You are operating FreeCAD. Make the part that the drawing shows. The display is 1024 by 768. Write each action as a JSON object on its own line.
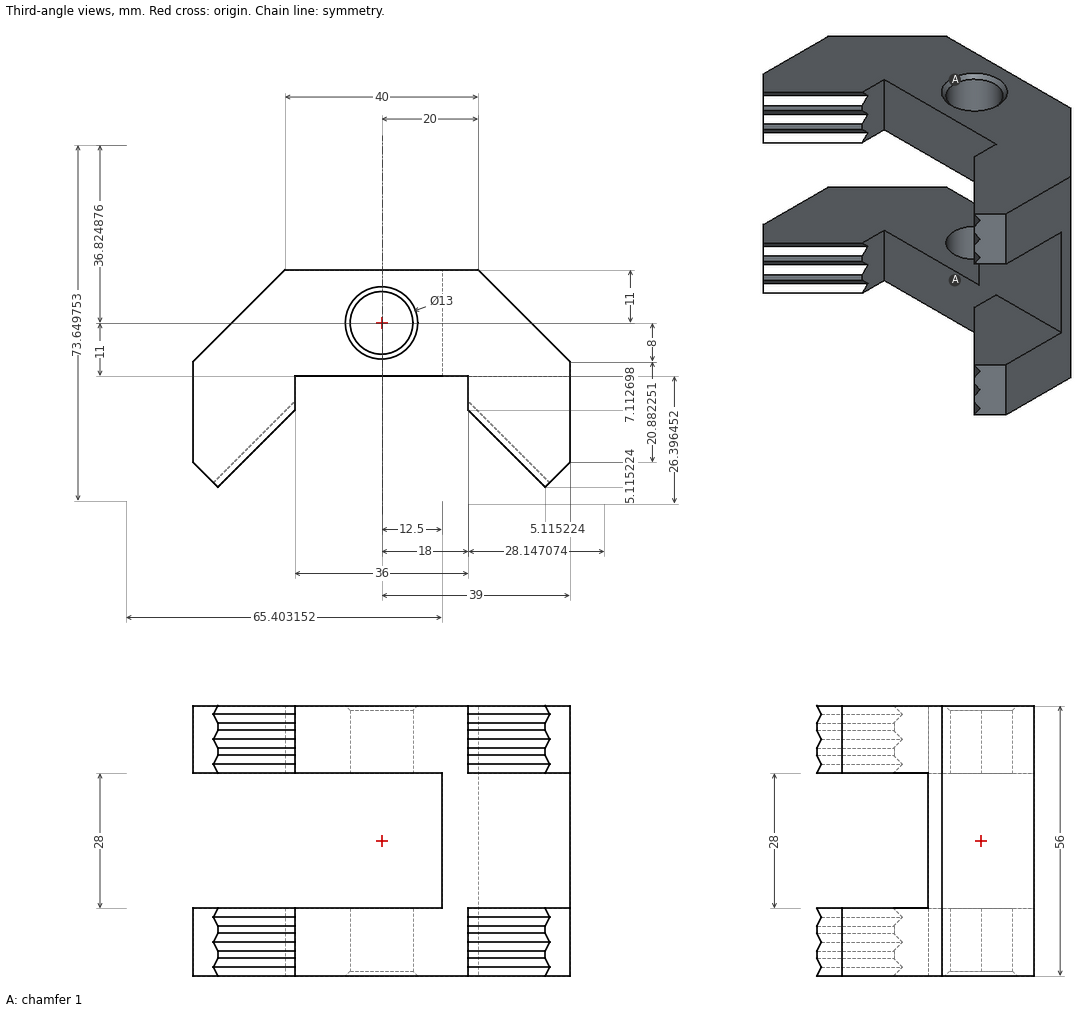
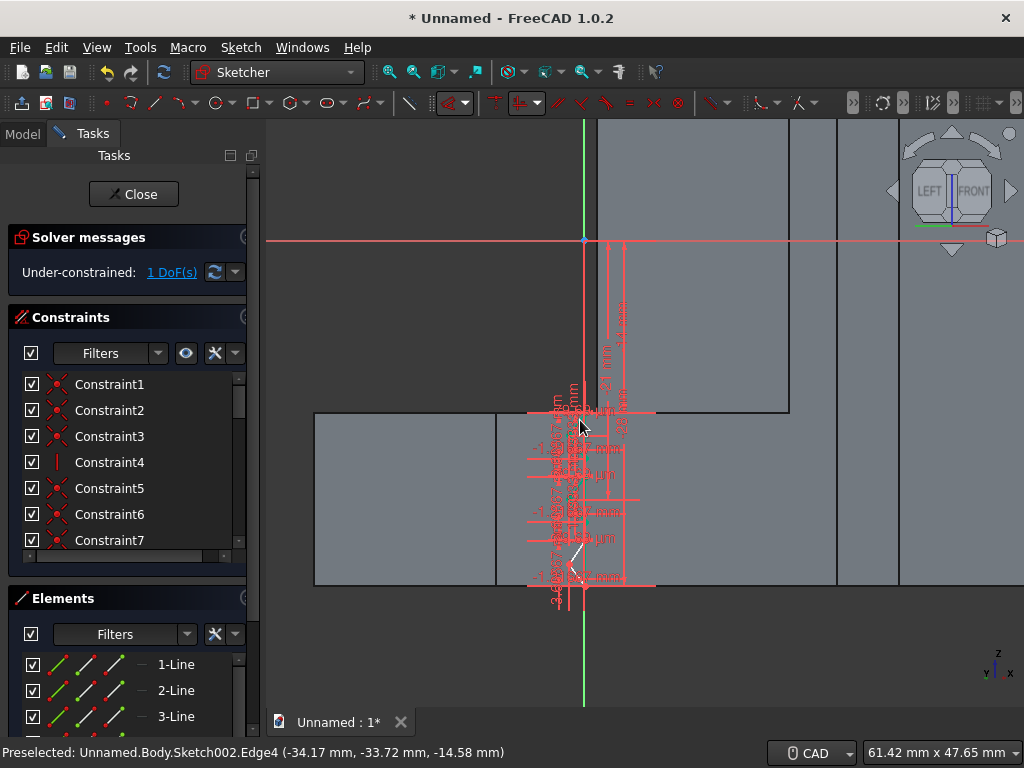
{"action": "scroll", "coordinate": [580, 548], "scroll_direction": "up", "scroll_amount": 7}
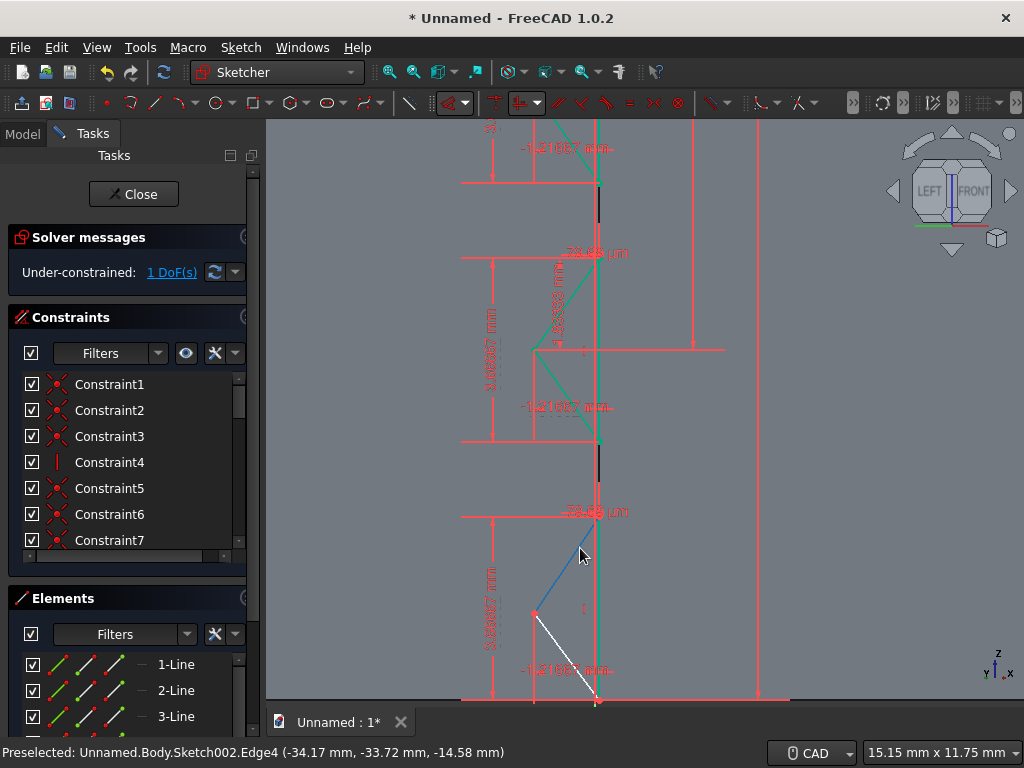
{"action": "left_click", "coordinate": [580, 546]}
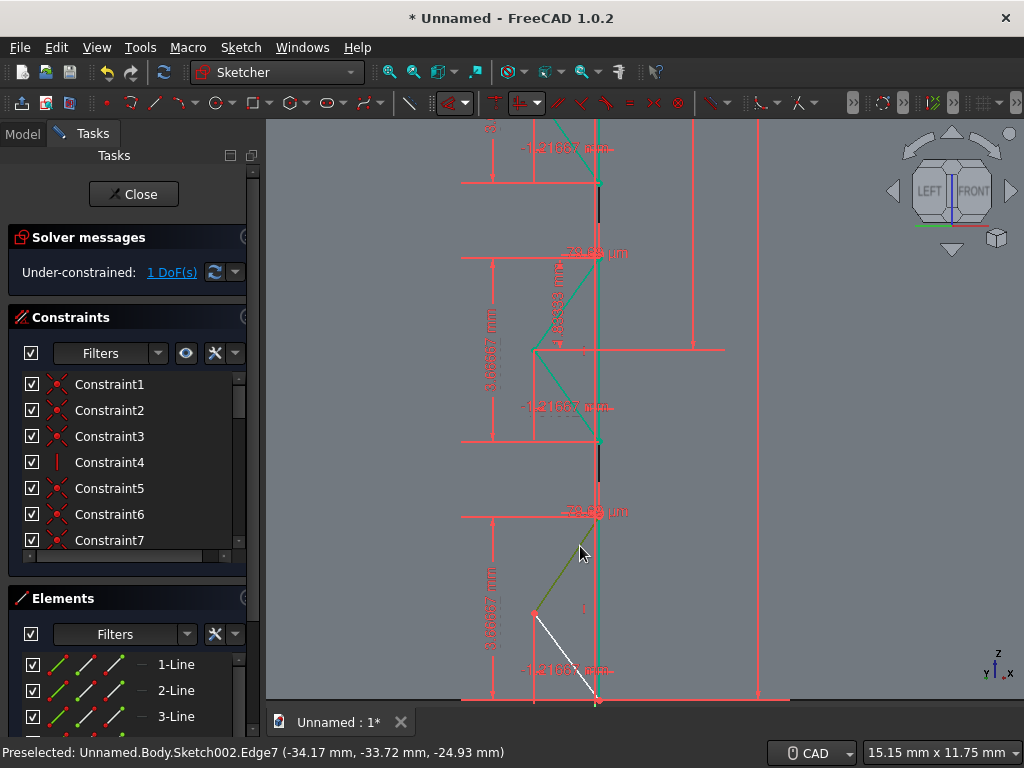
{"action": "left_click", "coordinate": [468, 104]}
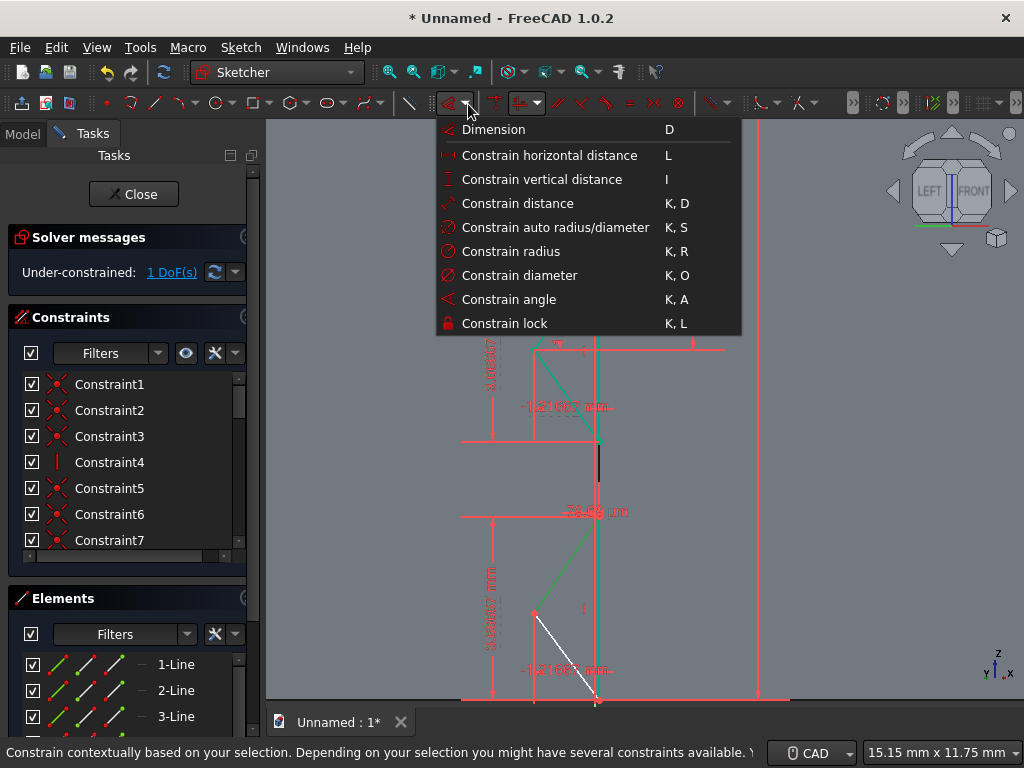
{"action": "left_click", "coordinate": [589, 179]}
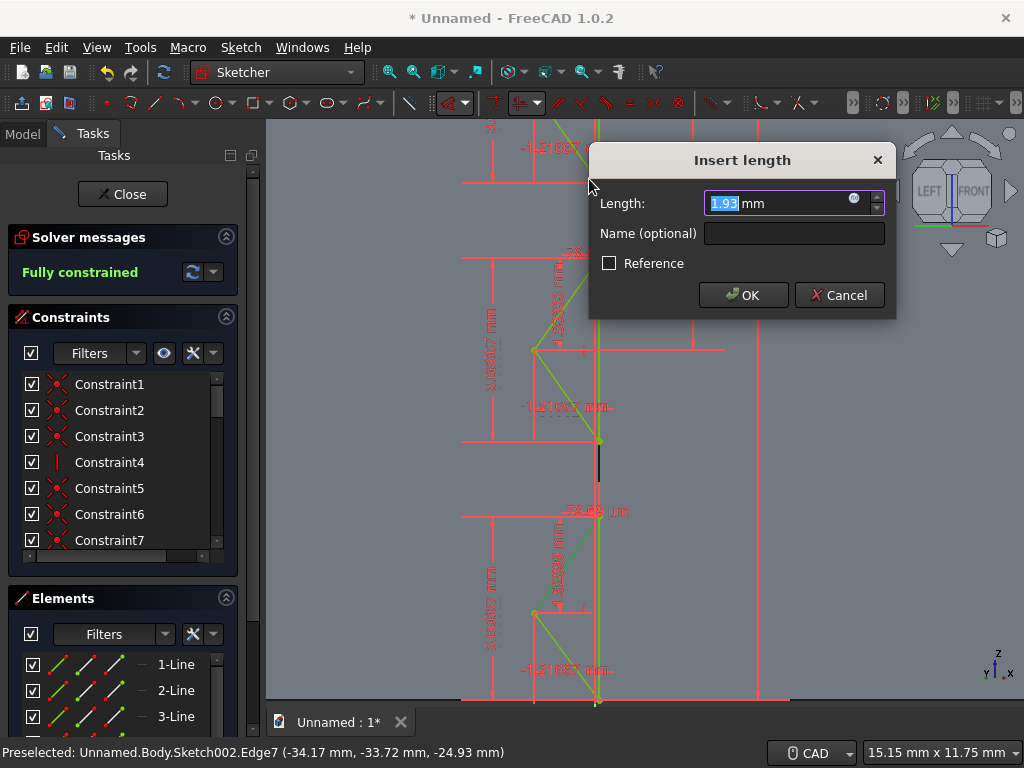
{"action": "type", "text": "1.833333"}
{"action": "key", "text": "Return"}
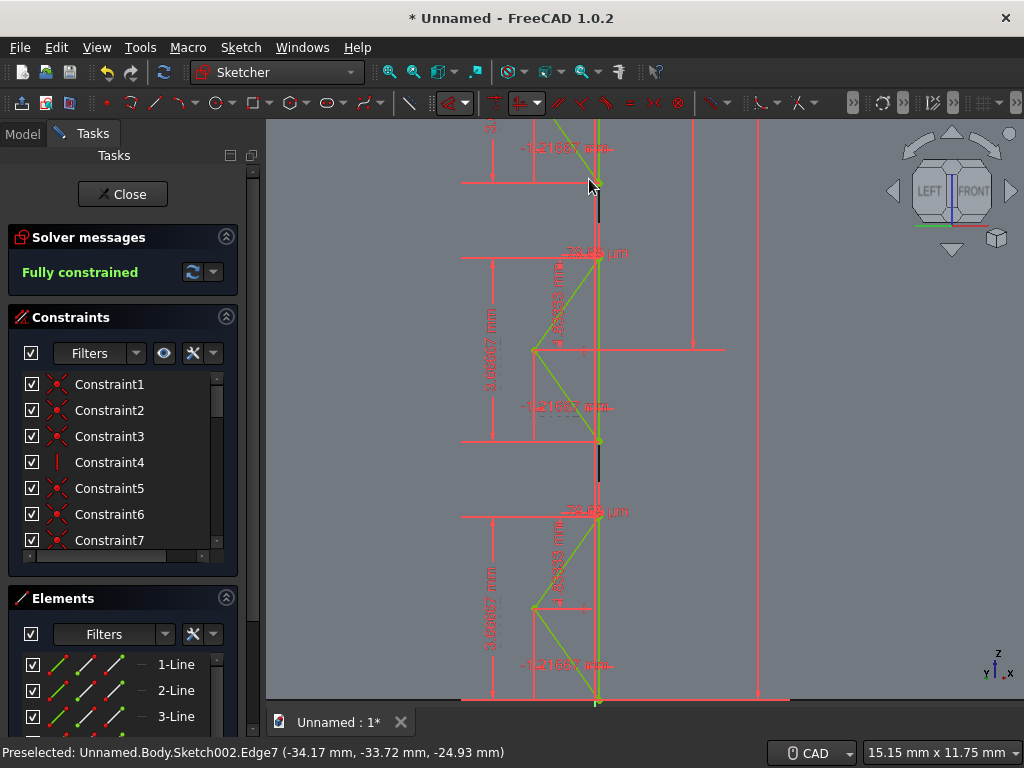
{"action": "left_click", "coordinate": [123, 194]}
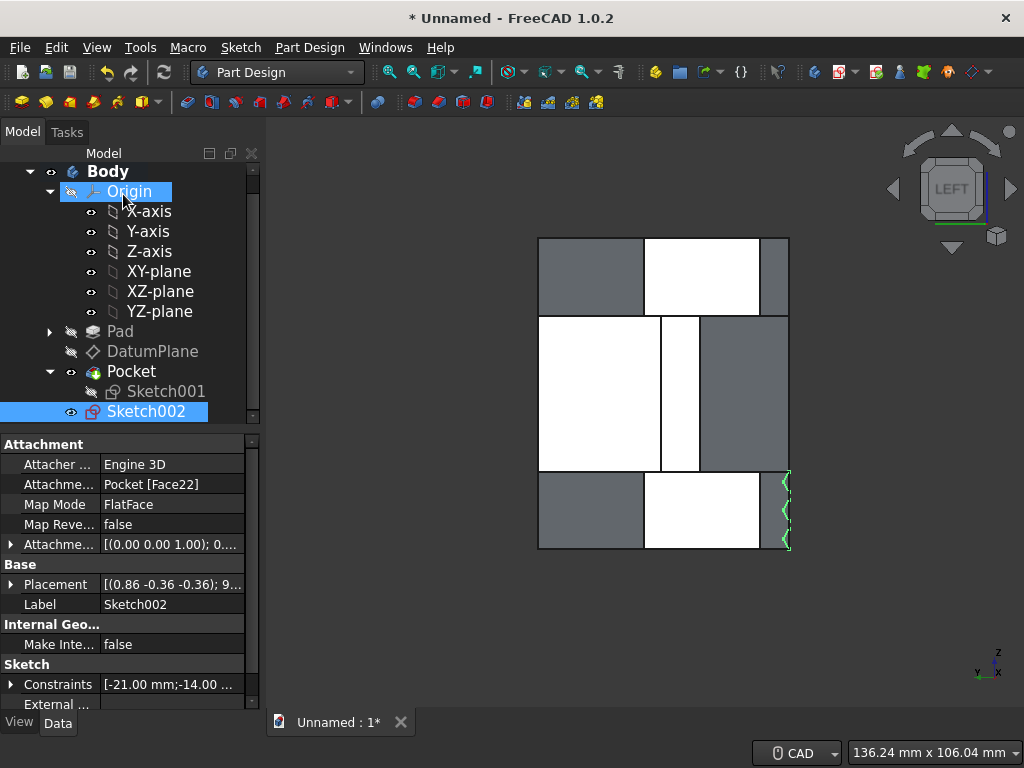
{"action": "left_click", "coordinate": [188, 102]}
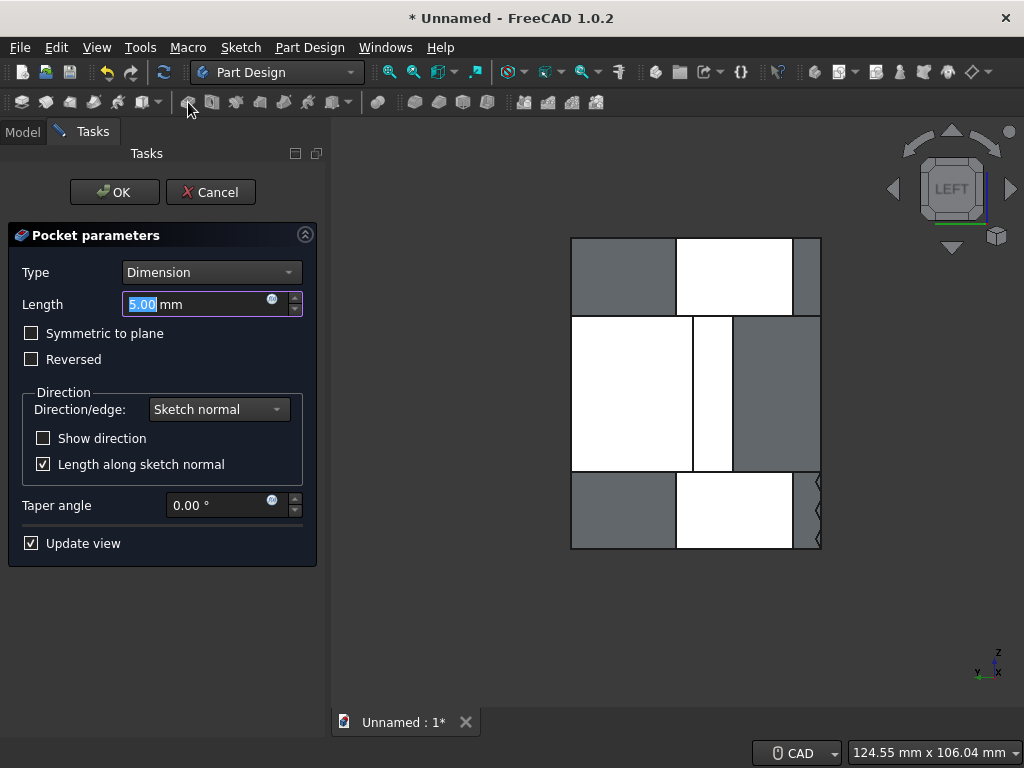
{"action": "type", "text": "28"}
{"action": "key", "text": "Tab"}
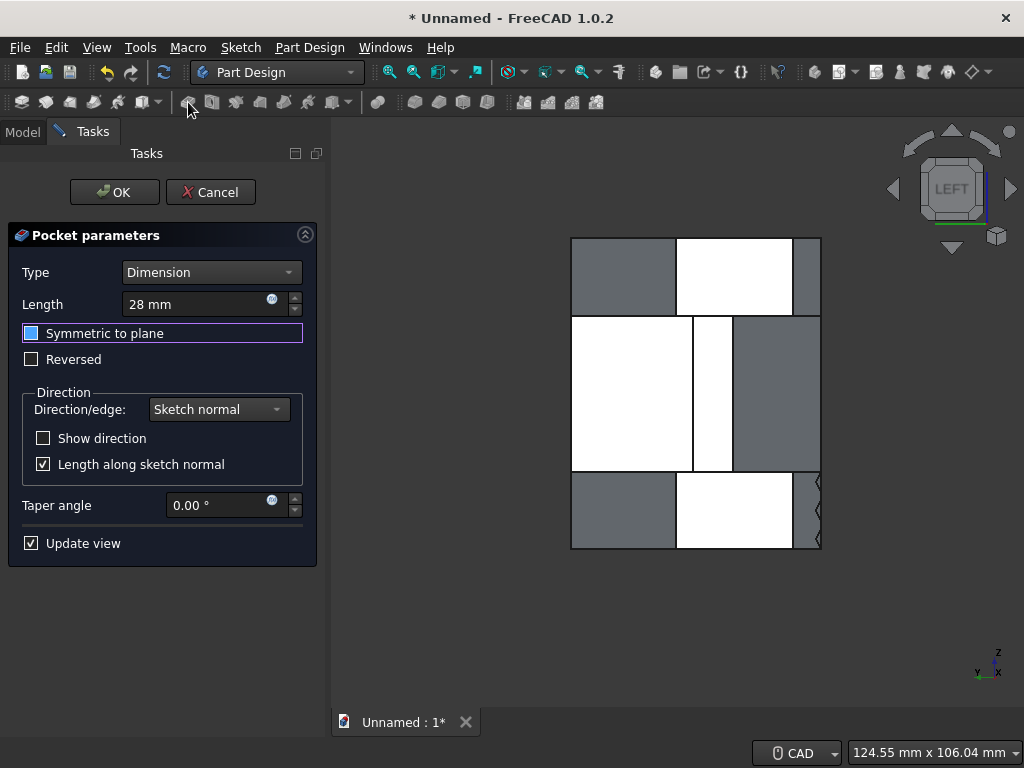
{"action": "left_click", "coordinate": [115, 192]}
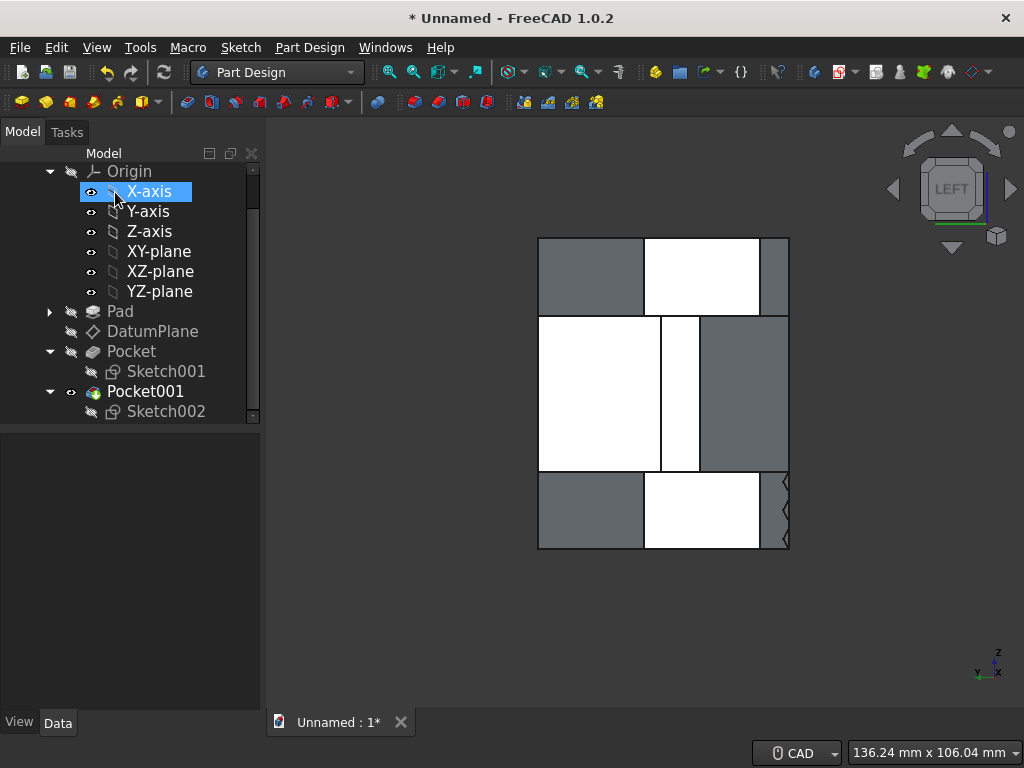
{"action": "left_click", "coordinate": [116, 392]}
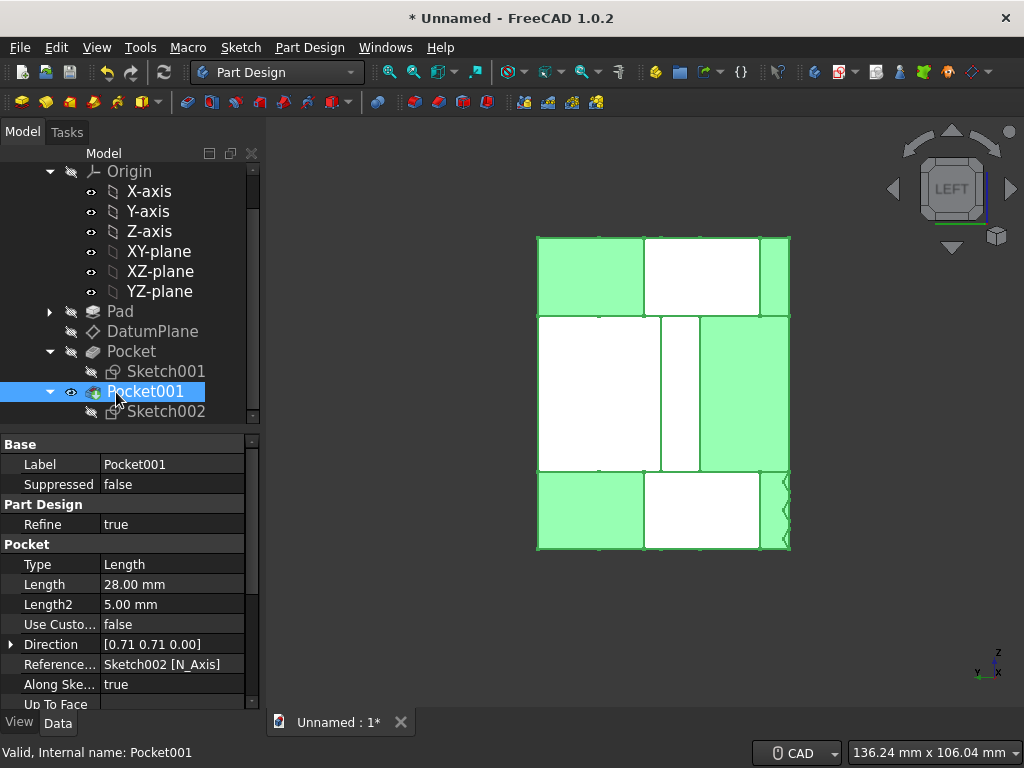
{"action": "left_click", "coordinate": [524, 102]}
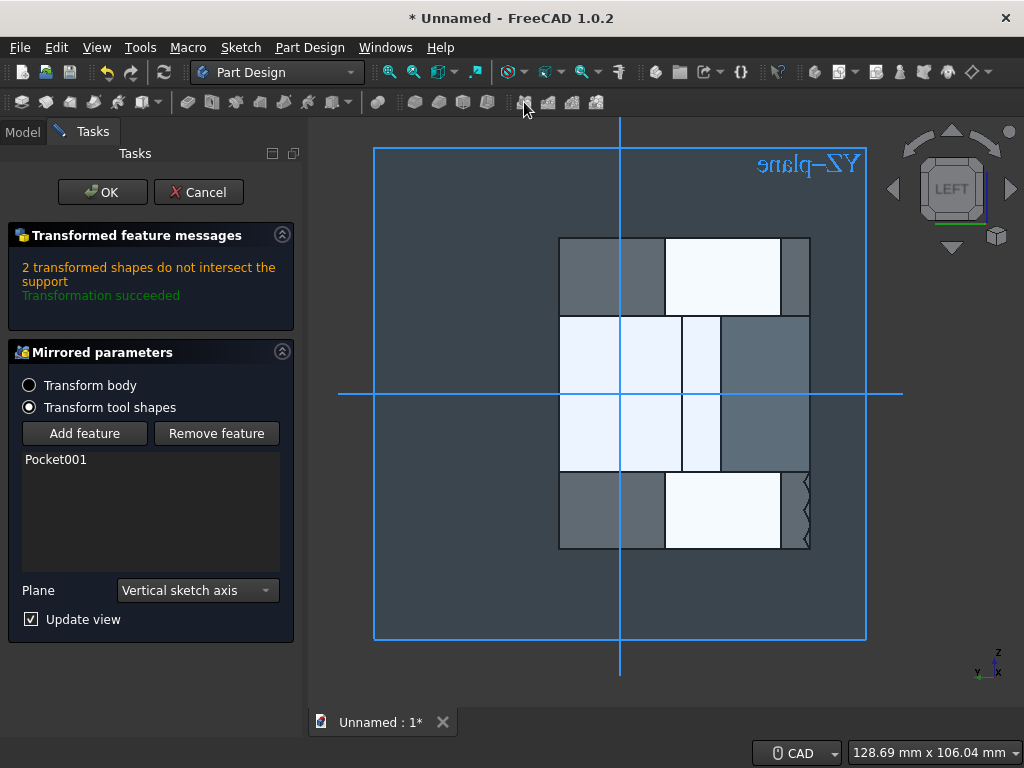
{"action": "left_click", "coordinate": [198, 590]}